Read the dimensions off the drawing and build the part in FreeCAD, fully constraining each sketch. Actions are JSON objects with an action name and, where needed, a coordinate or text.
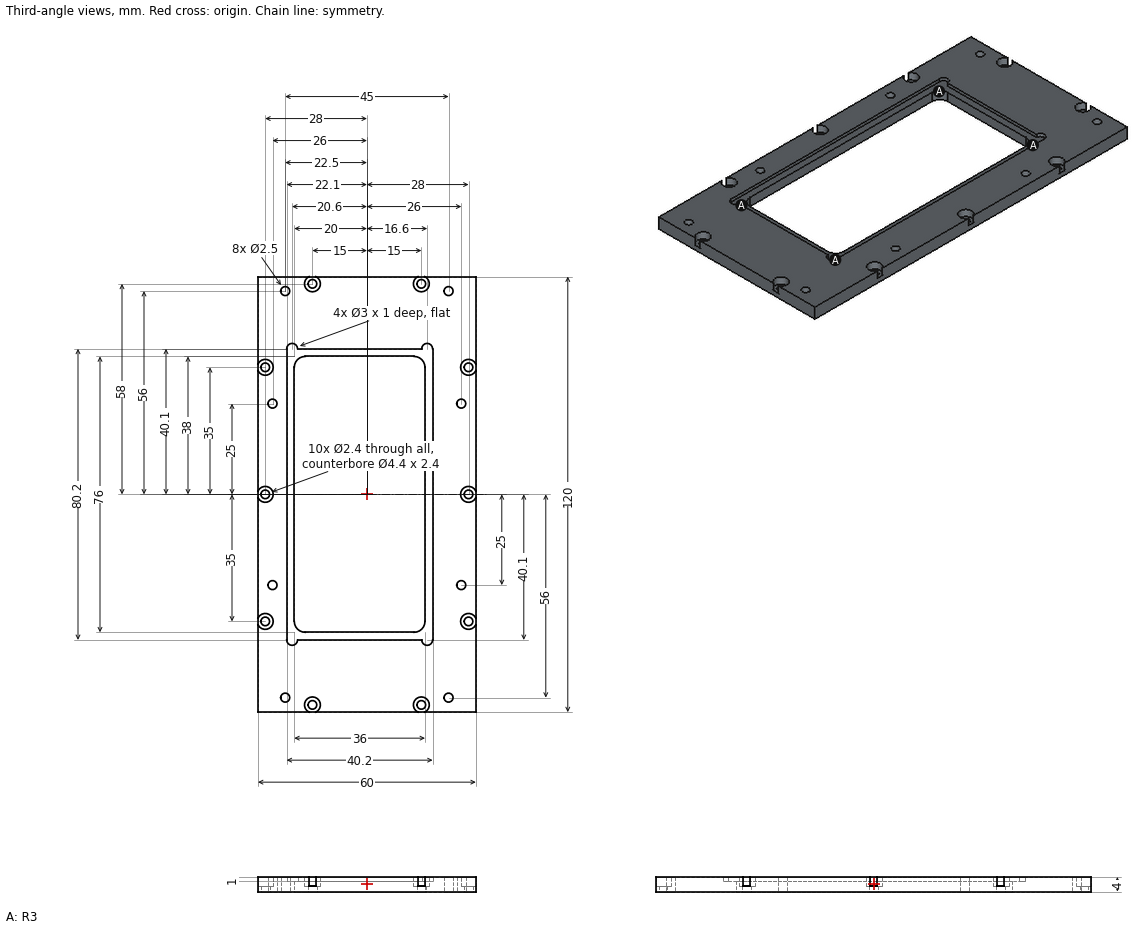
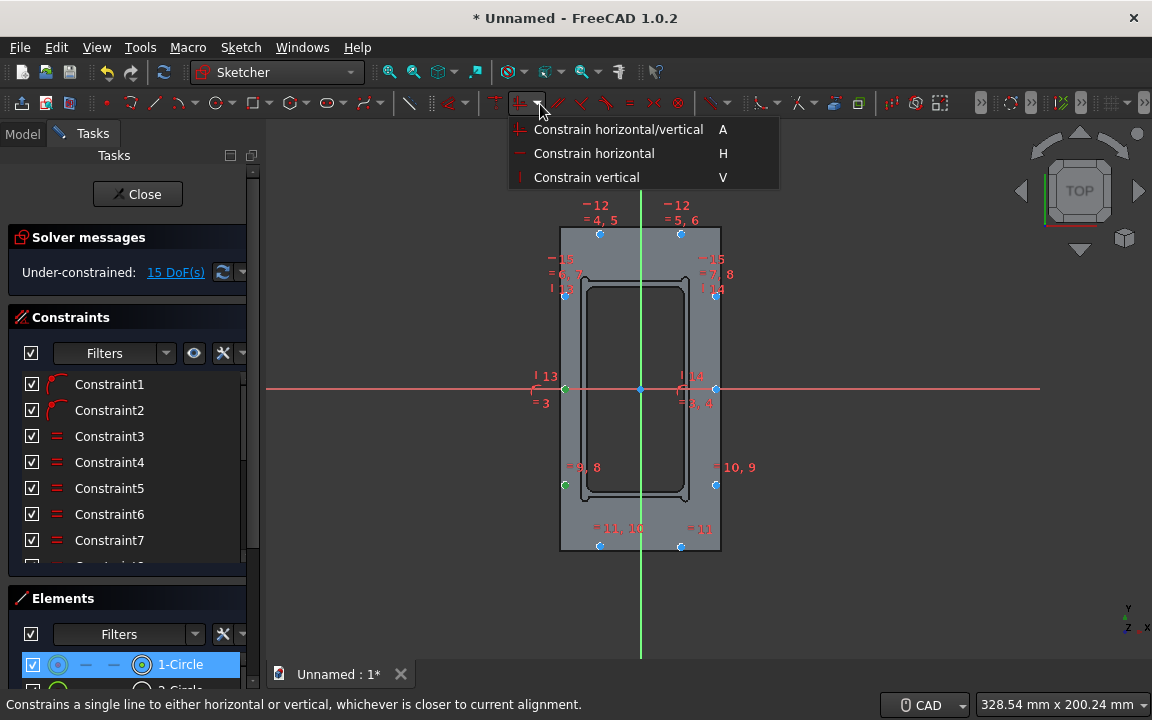
{"action": "left_click", "coordinate": [644, 177]}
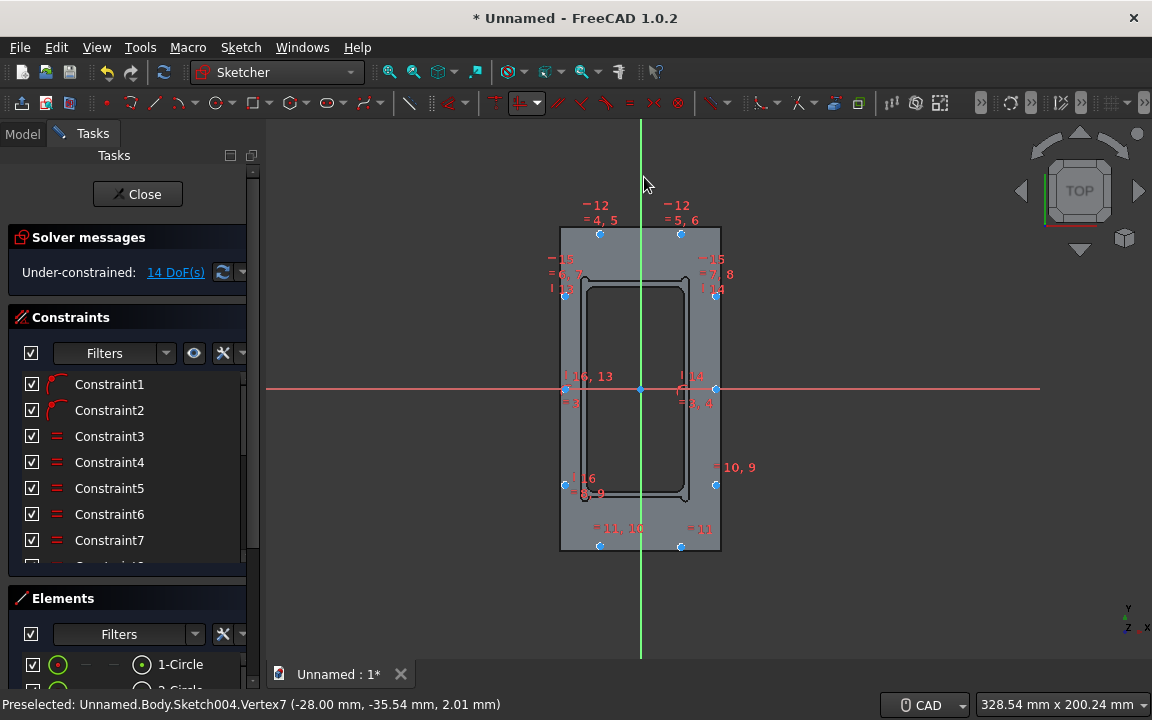
{"action": "left_click", "coordinate": [716, 389]}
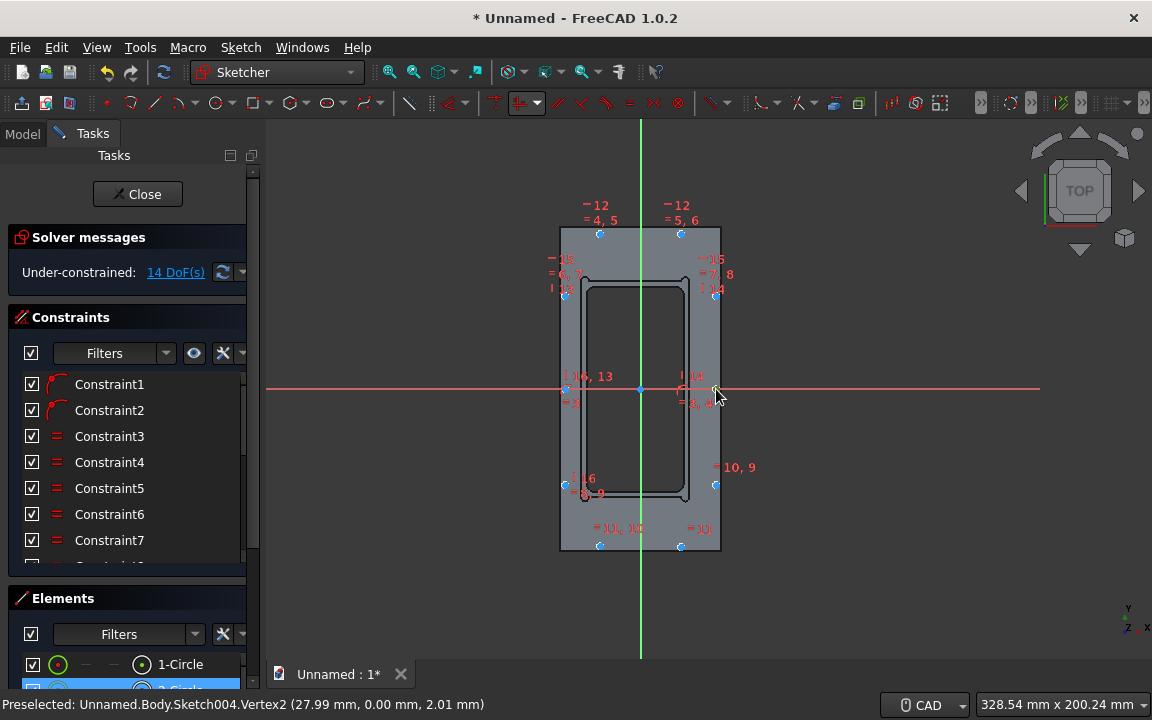
{"action": "left_click", "coordinate": [716, 485]}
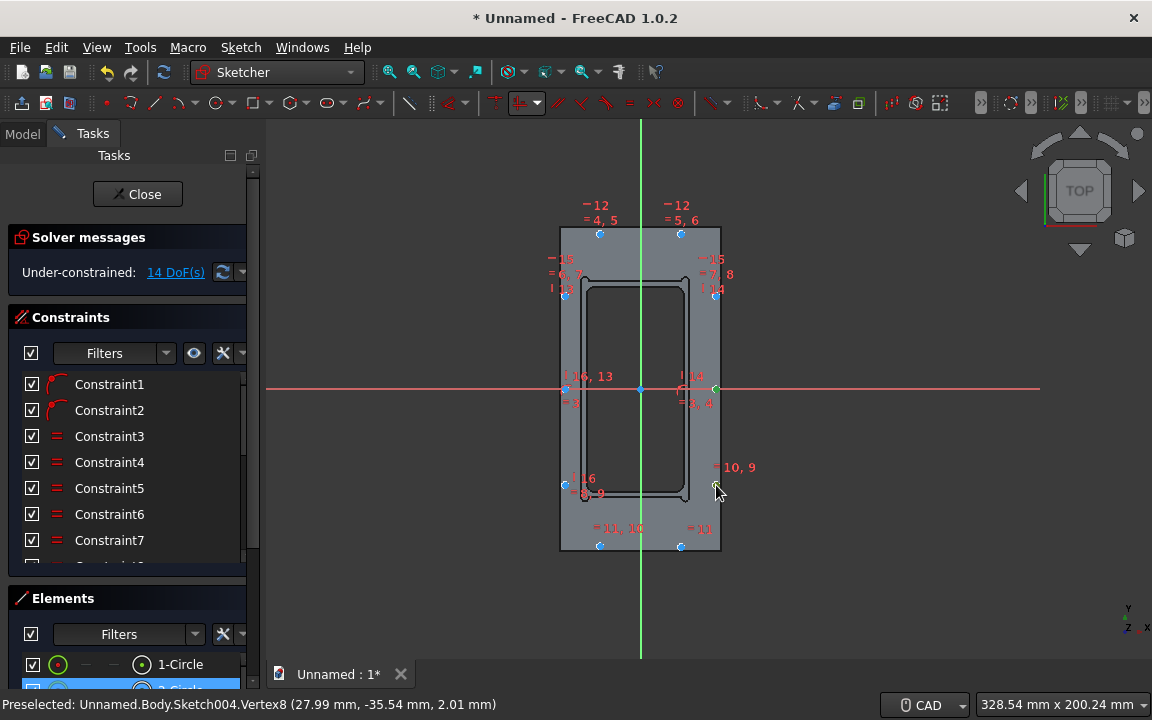
{"action": "key", "text": "v"}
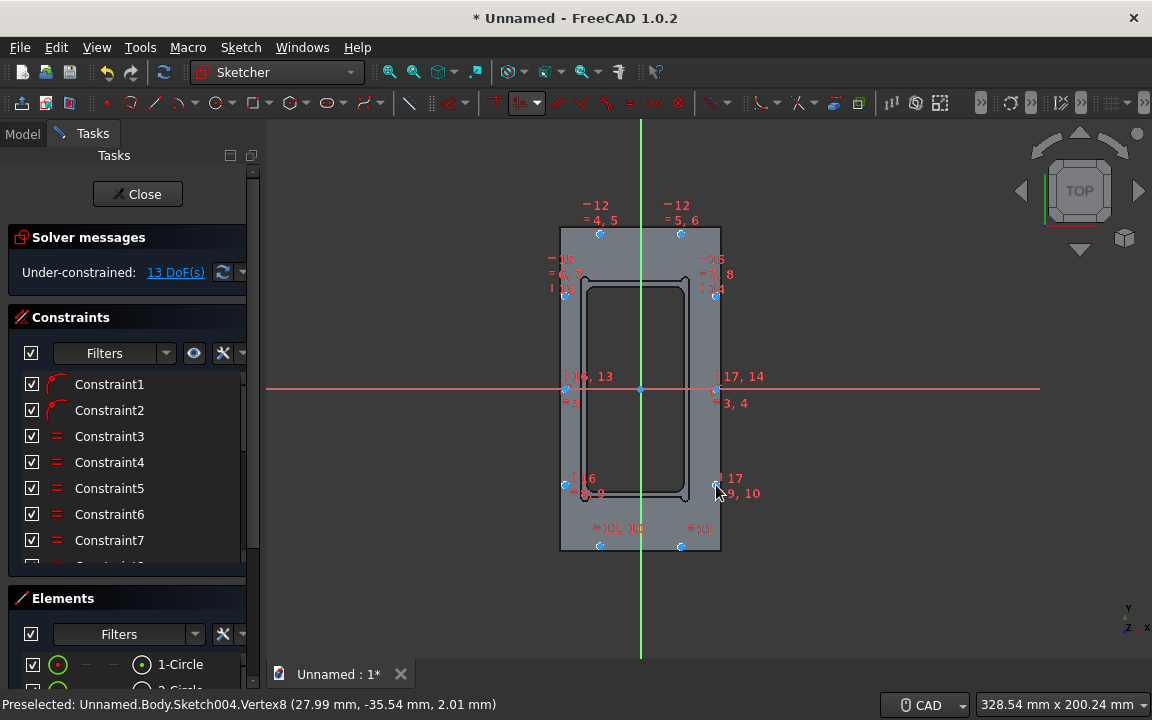
{"action": "left_click", "coordinate": [565, 485]}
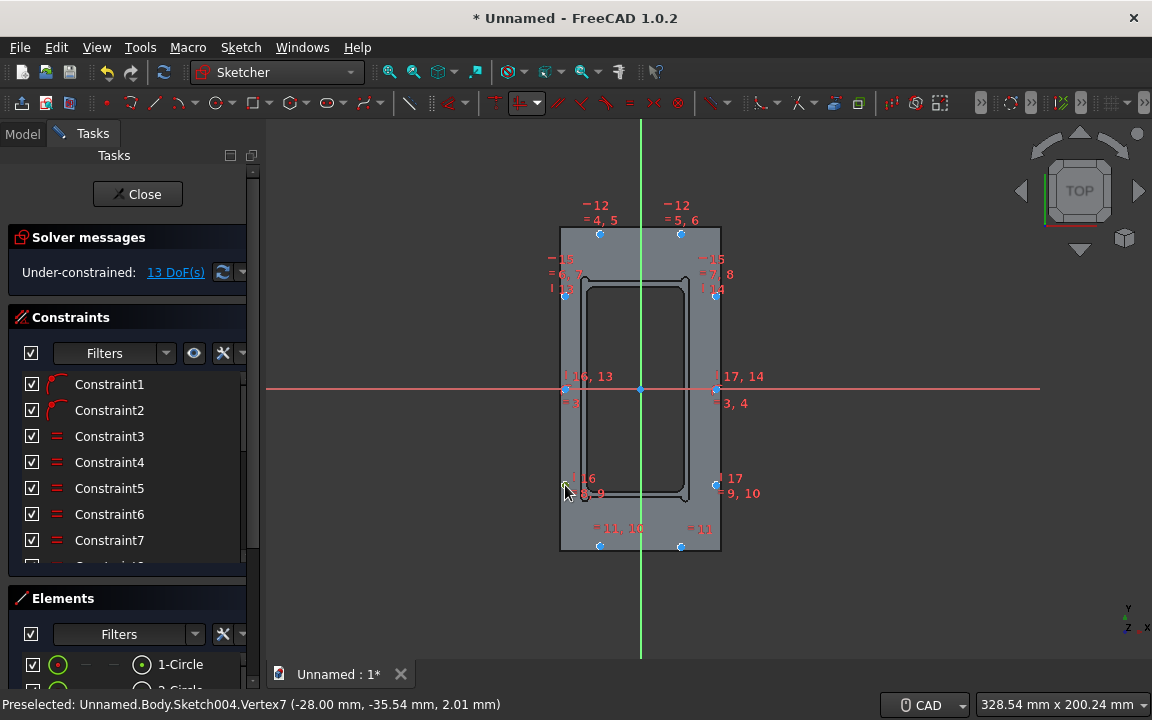
{"action": "left_click", "coordinate": [714, 487]}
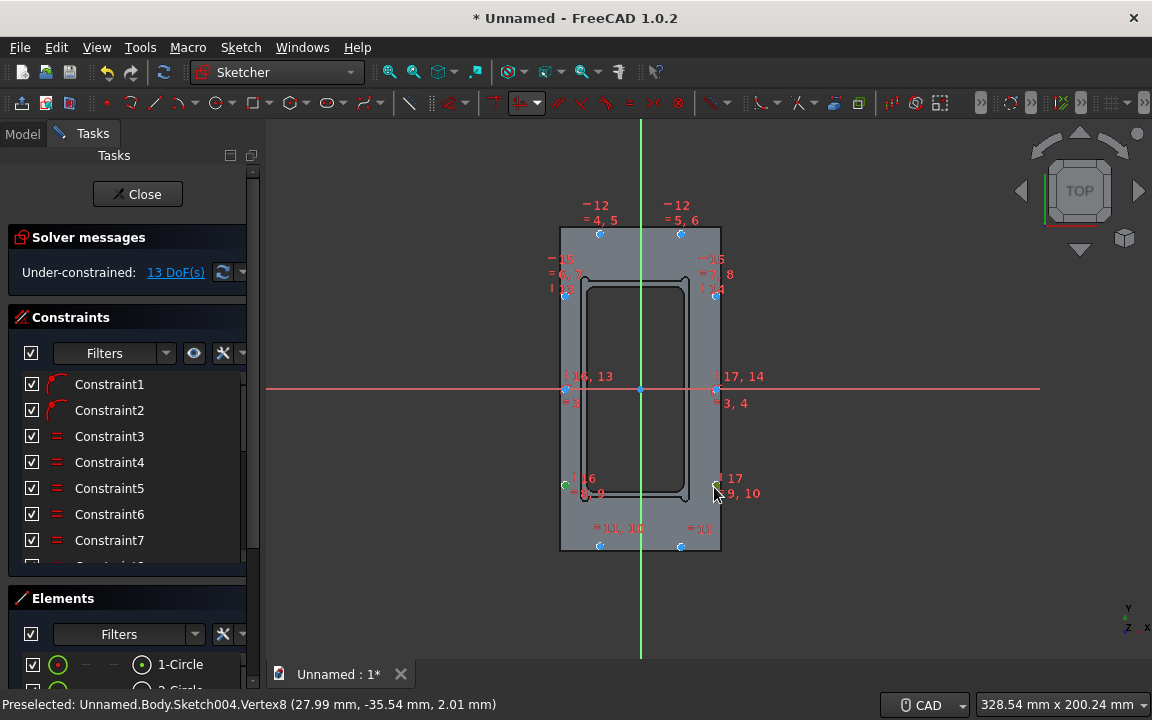
{"action": "key", "text": "h"}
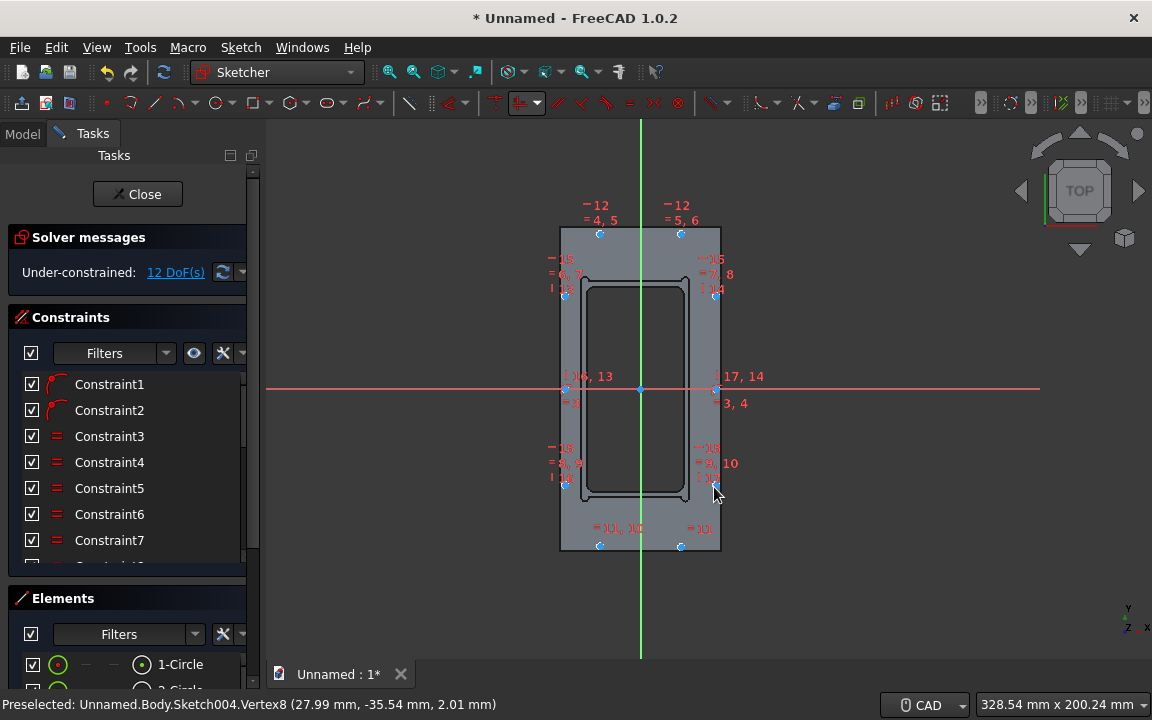
{"action": "left_click", "coordinate": [600, 546]}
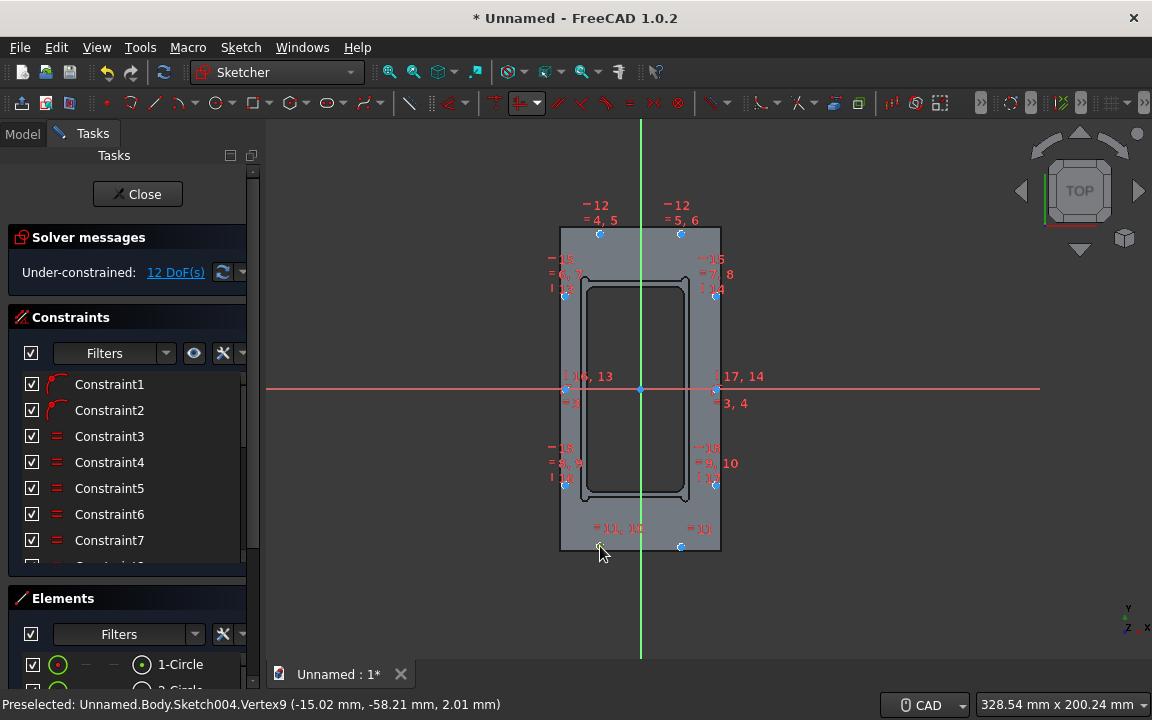
{"action": "left_click", "coordinate": [681, 547]}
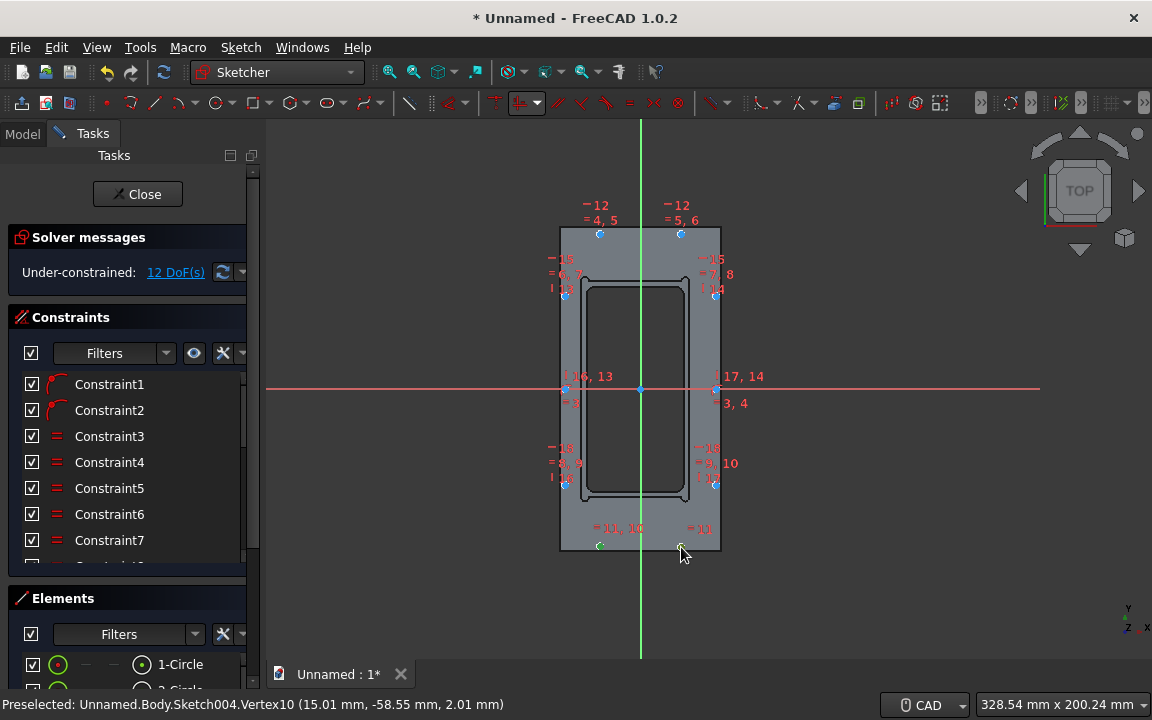
{"action": "key", "text": "h"}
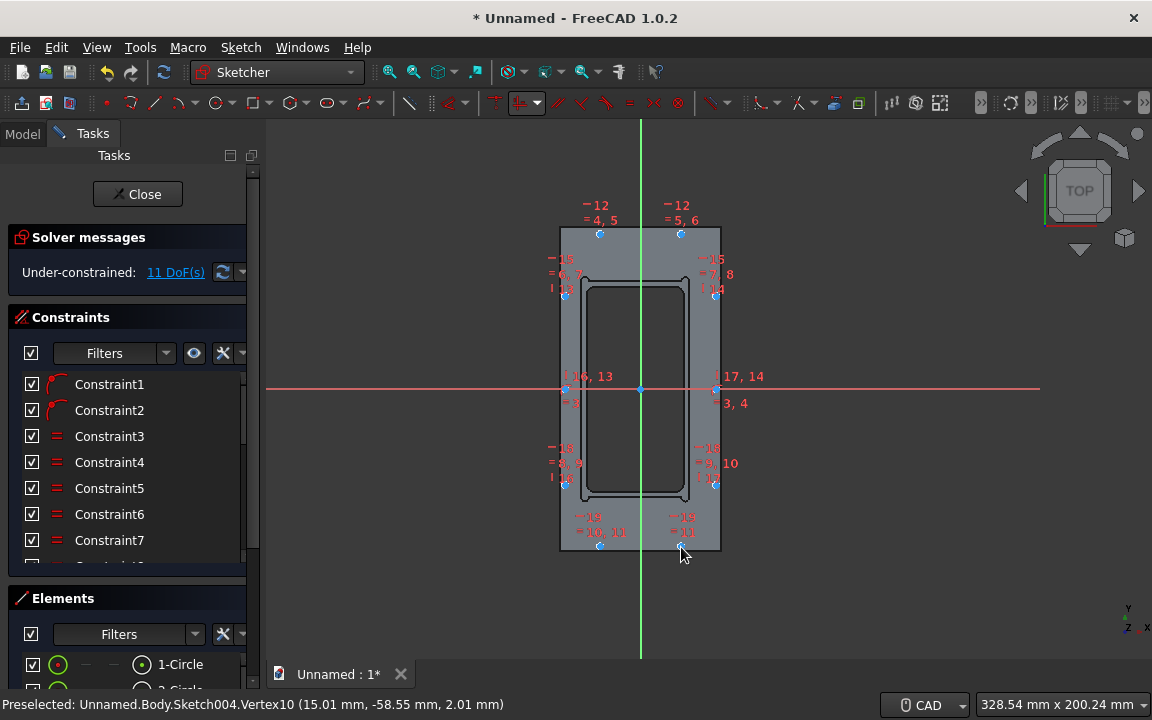
{"action": "left_click", "coordinate": [600, 234]}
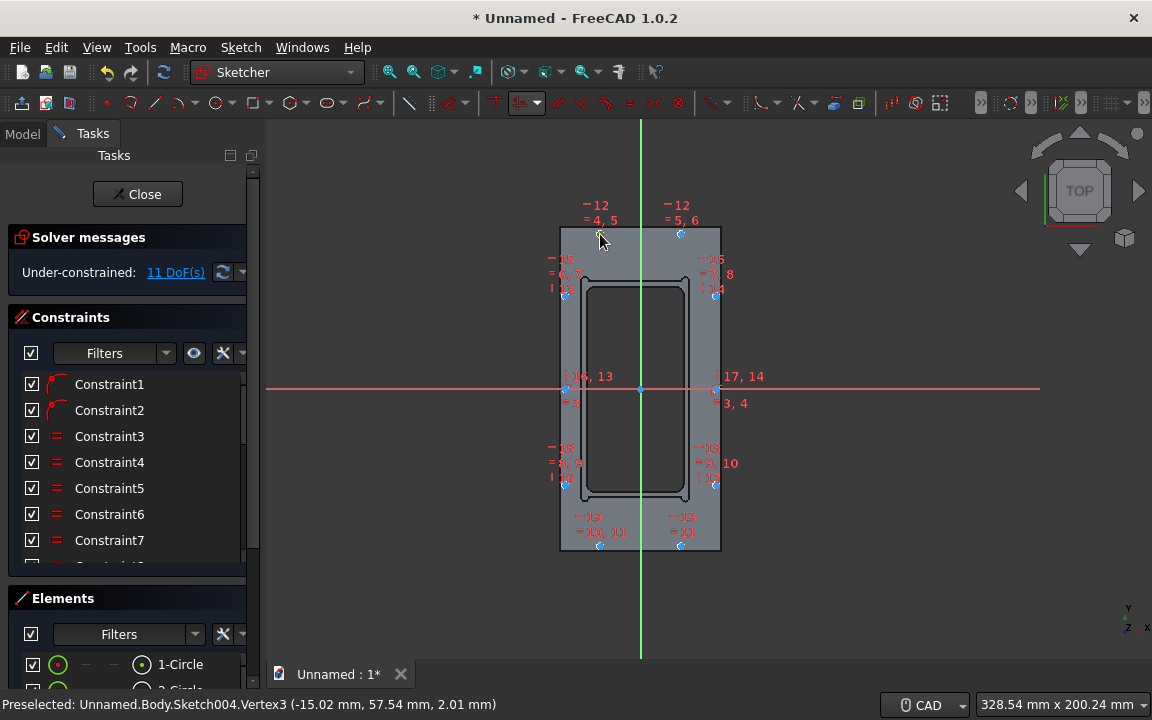
{"action": "left_click", "coordinate": [600, 546]}